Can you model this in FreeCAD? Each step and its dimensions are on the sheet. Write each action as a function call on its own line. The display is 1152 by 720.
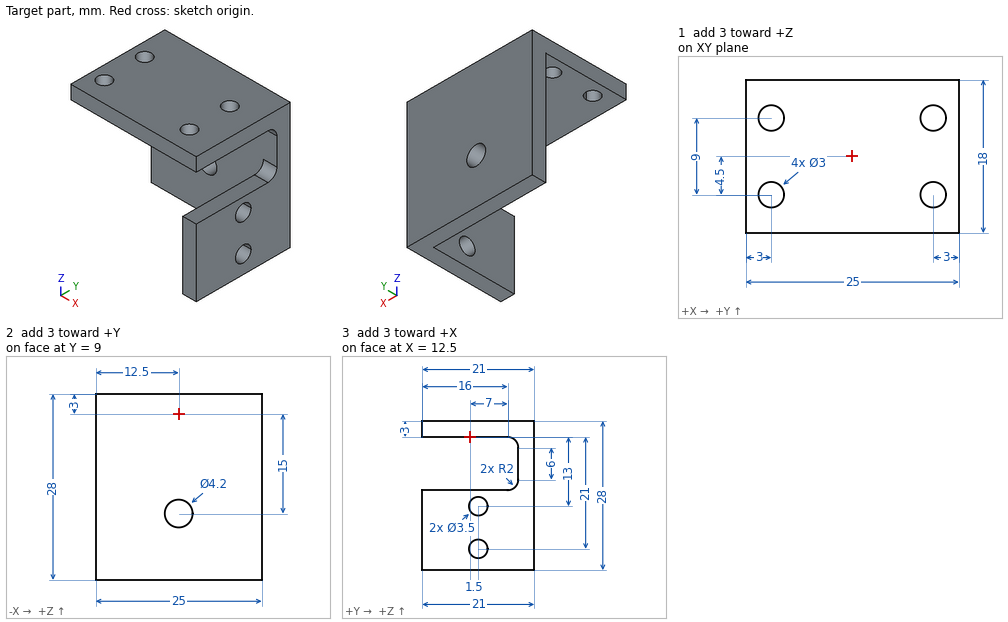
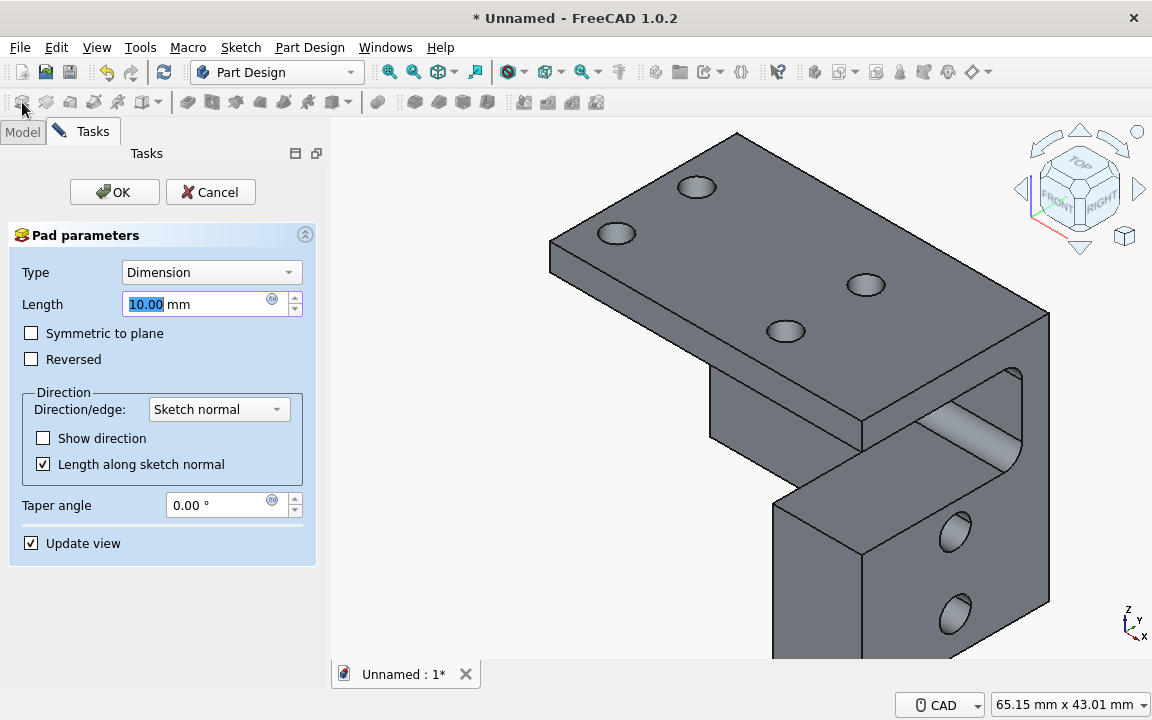
text(3)
key(Tab)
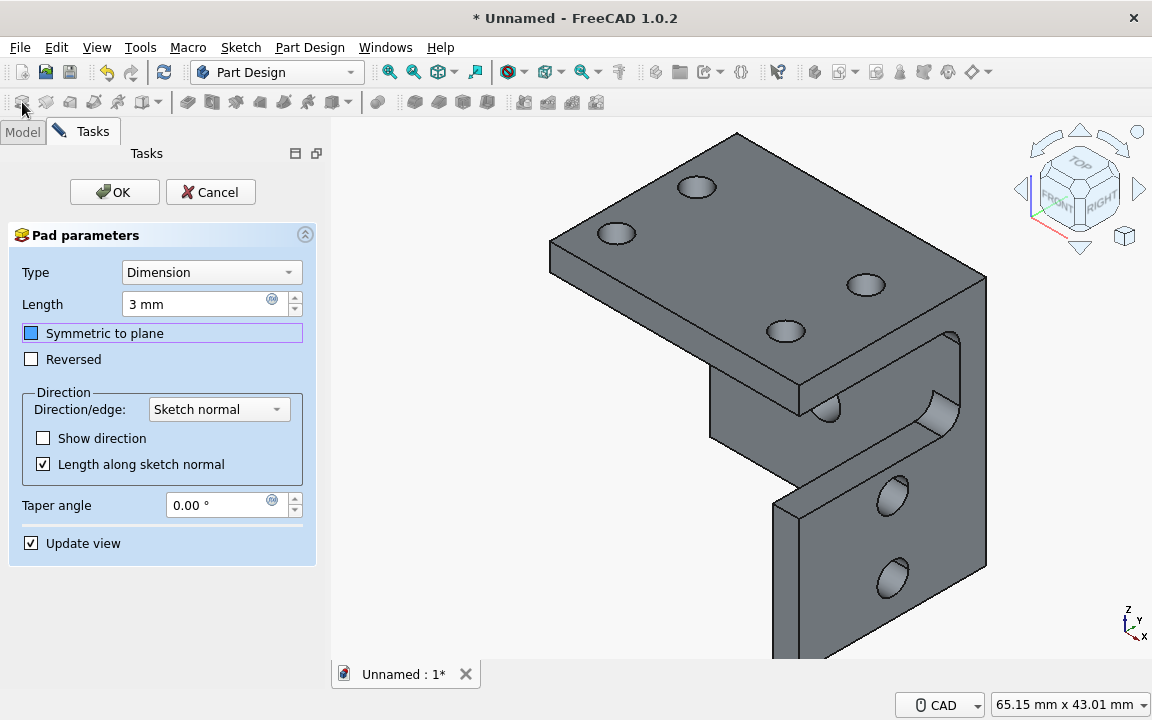
click(115, 192)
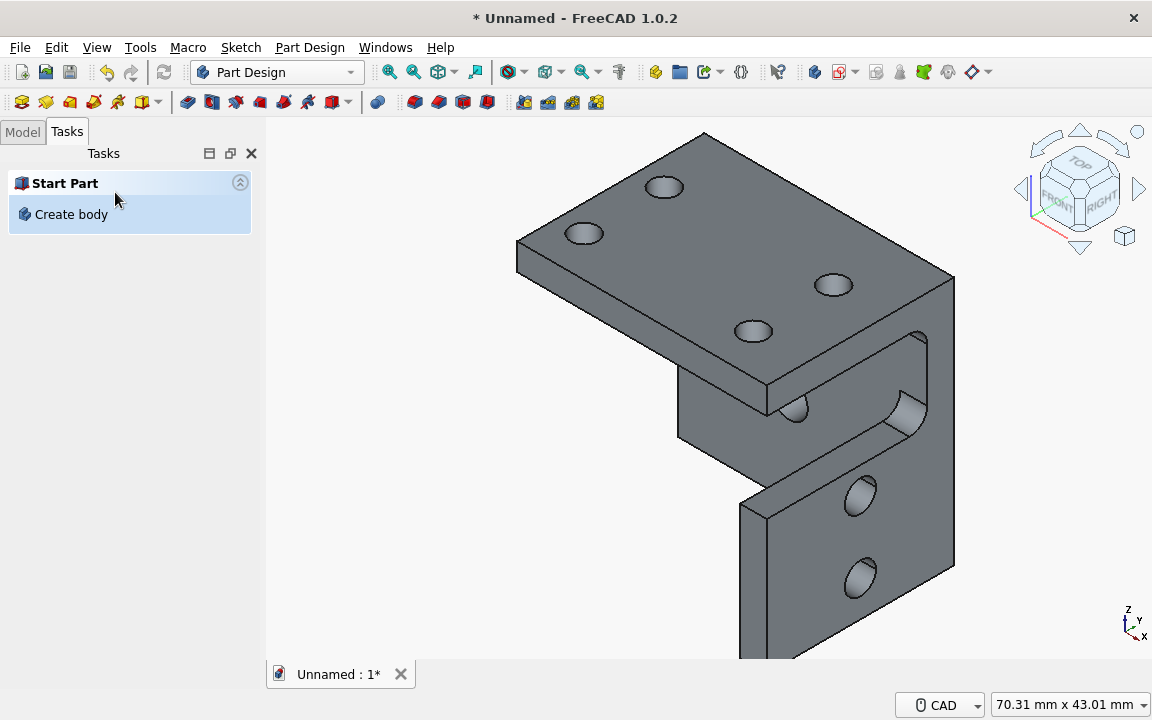
key(v)
key(f)